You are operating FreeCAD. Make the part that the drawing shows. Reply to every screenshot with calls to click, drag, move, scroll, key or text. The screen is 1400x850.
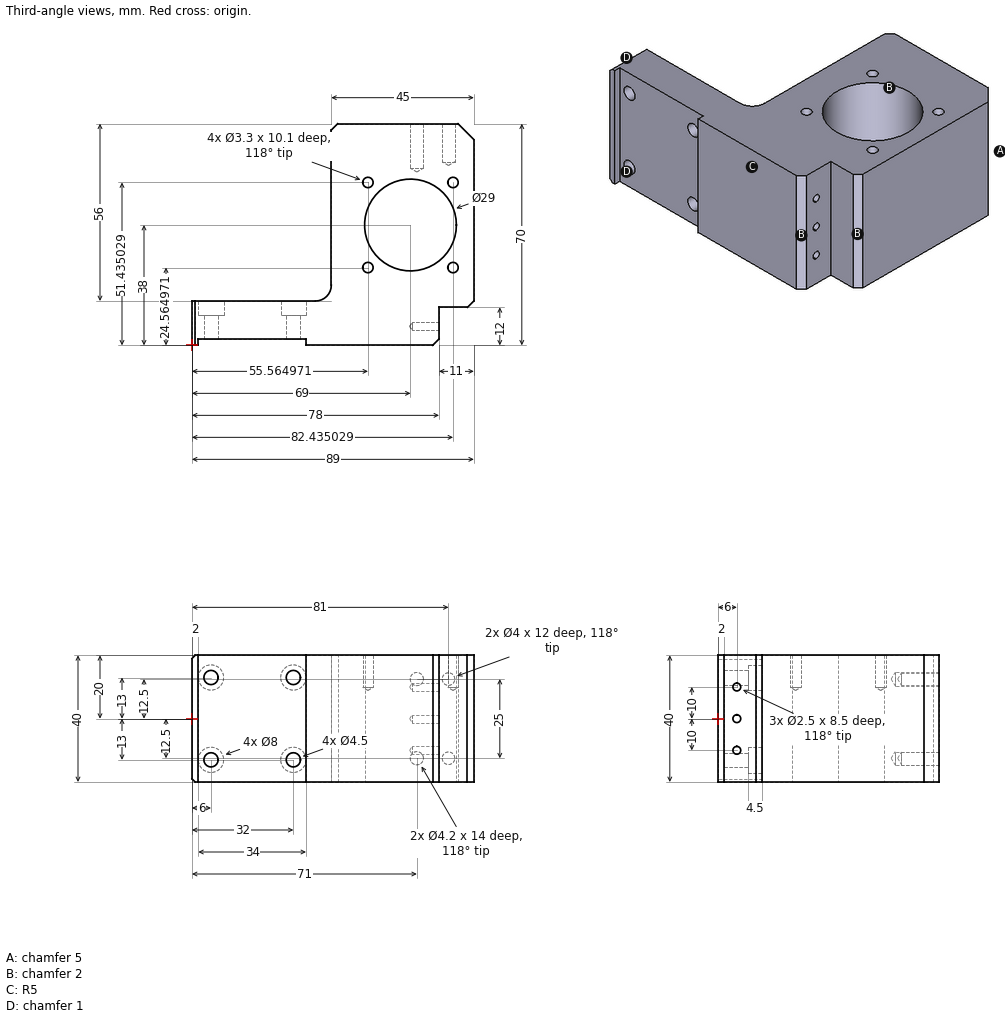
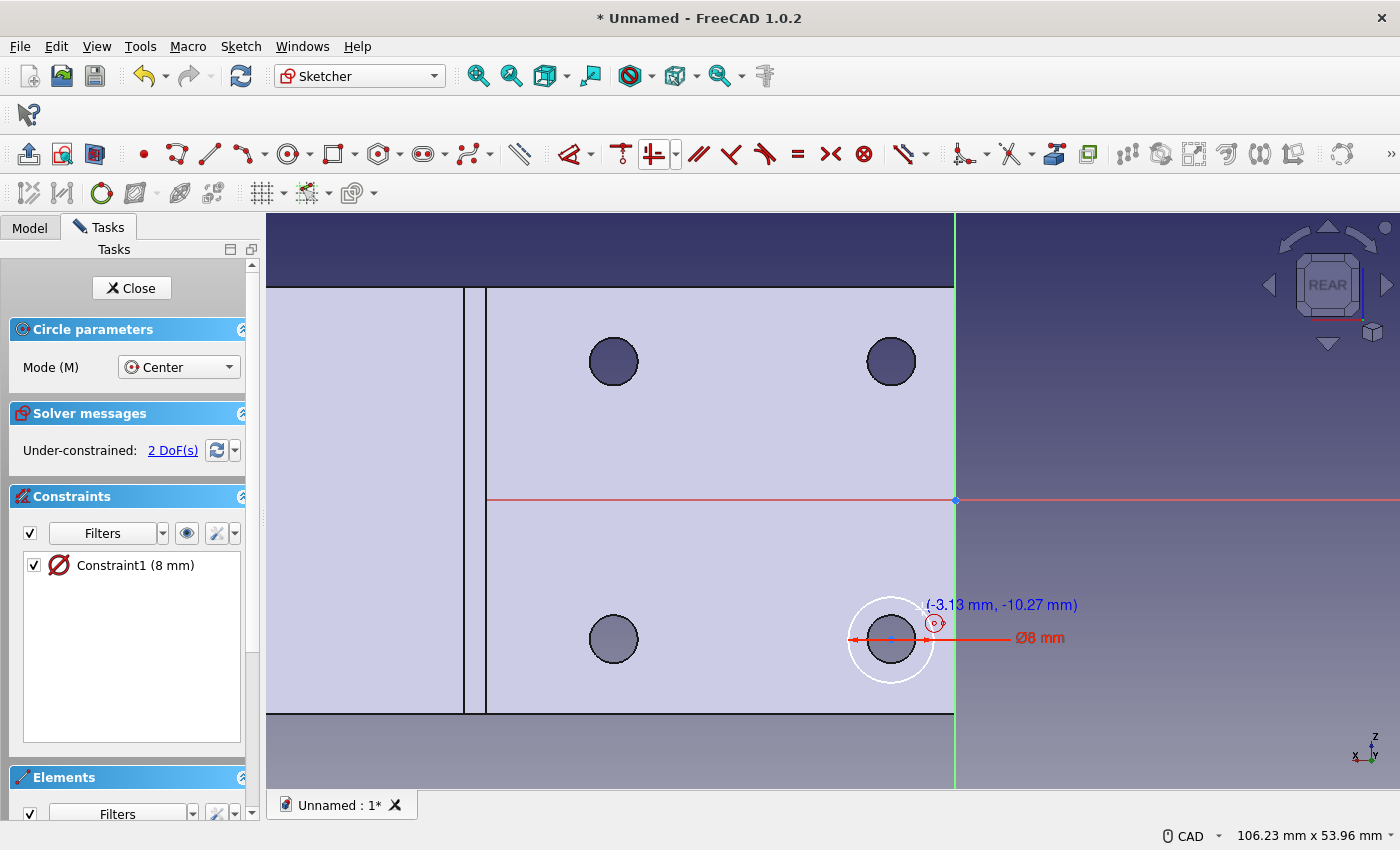
click(614, 639)
move(644, 609)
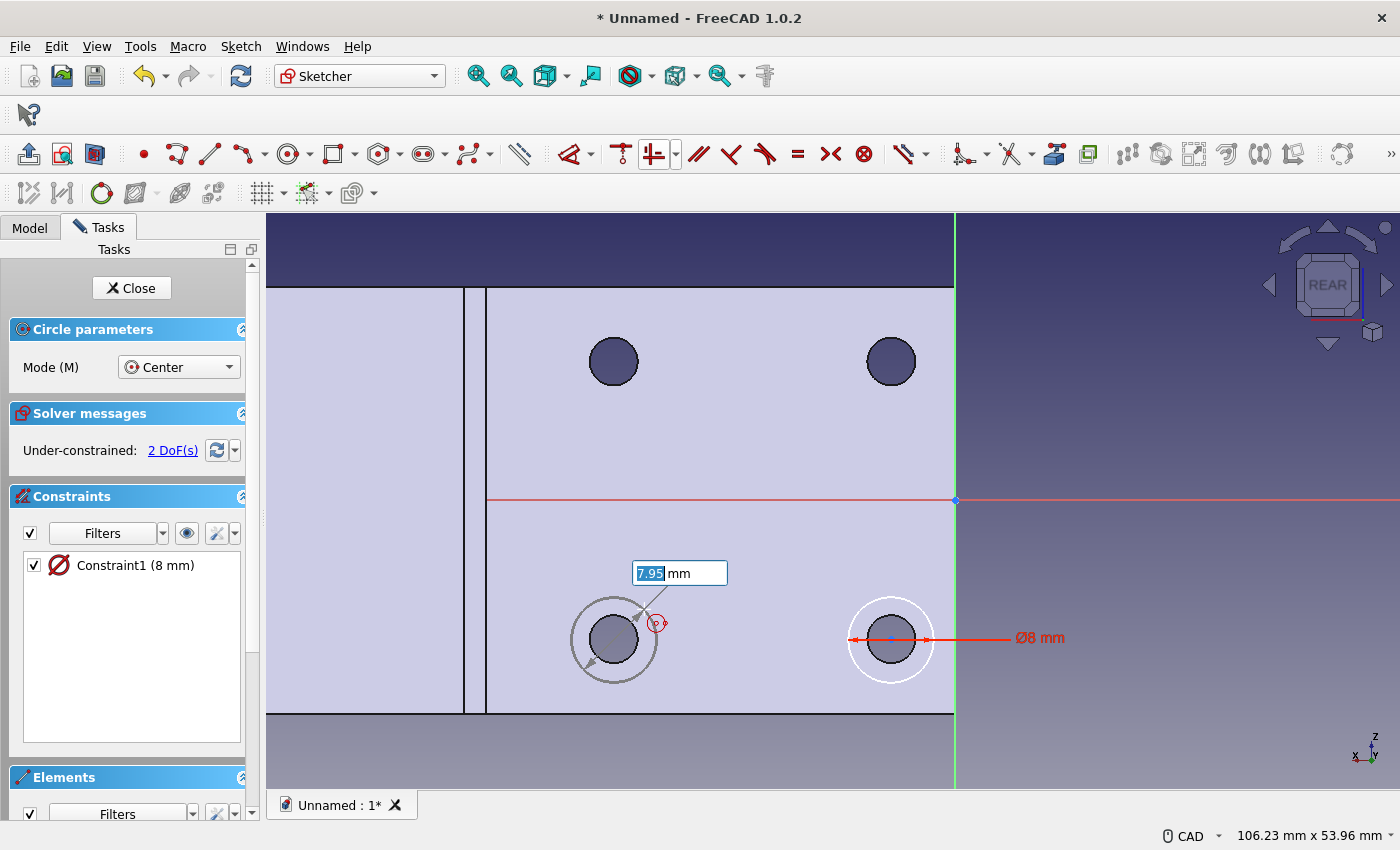
text(8)
key(Return)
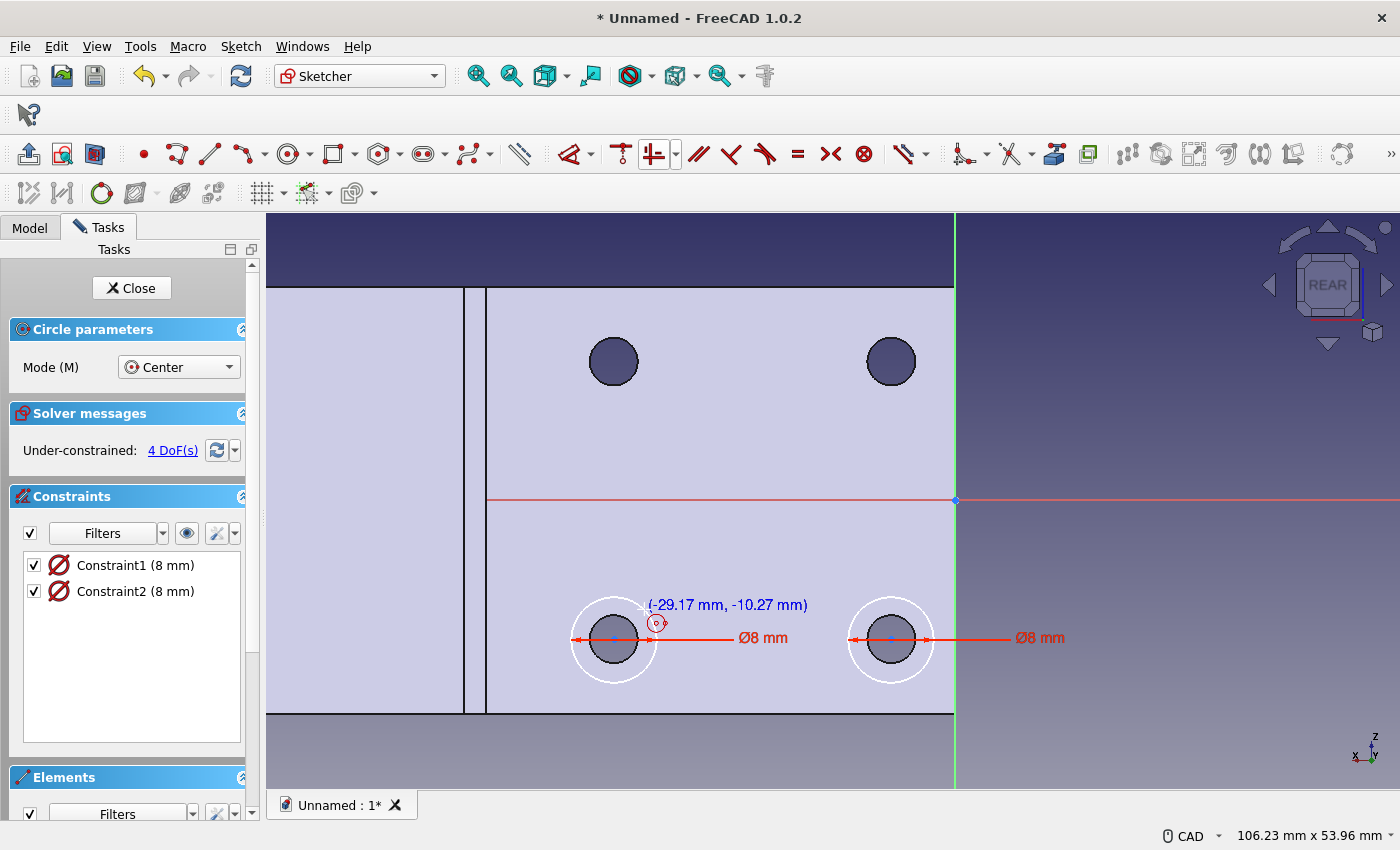
click(614, 362)
move(644, 331)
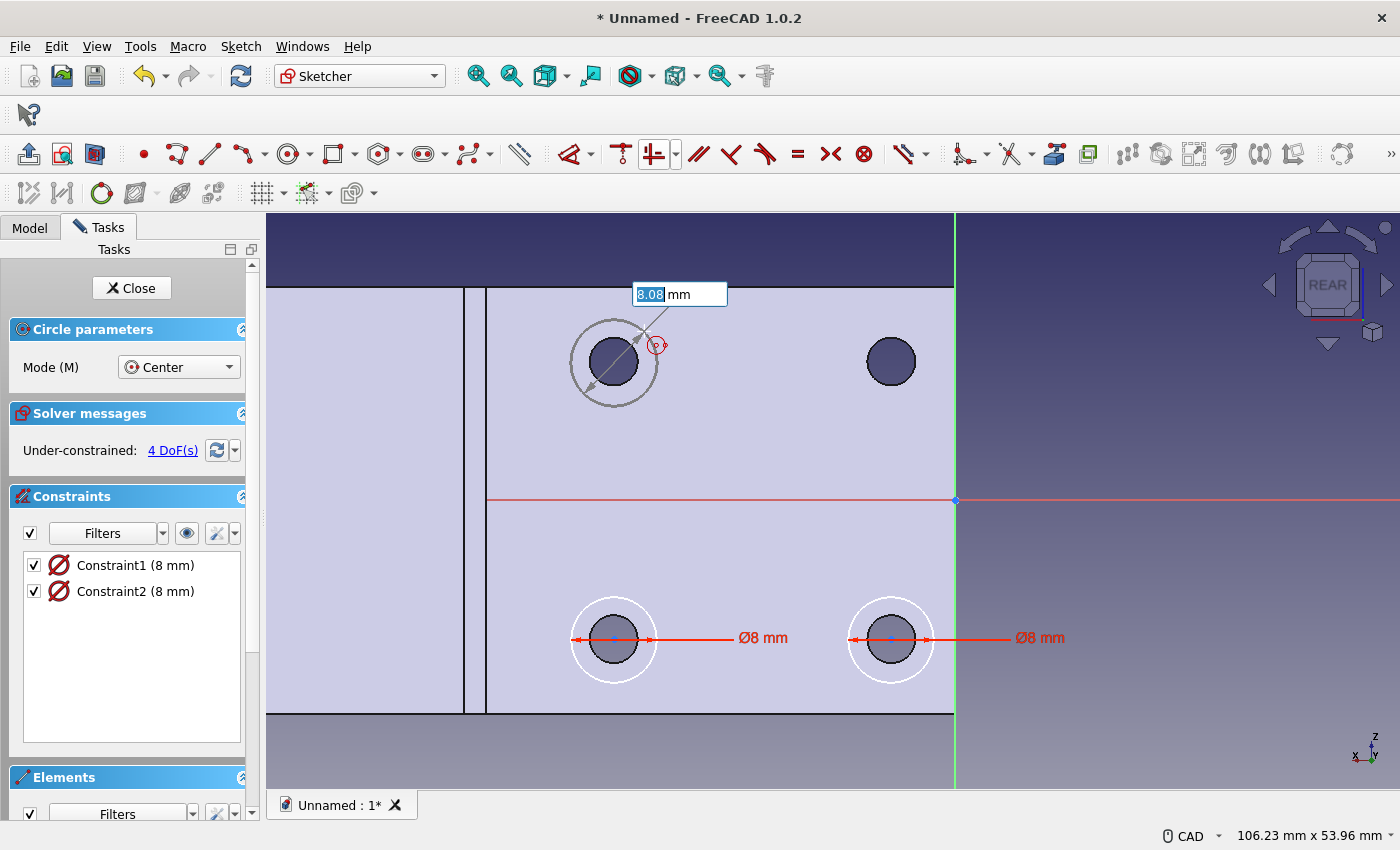
text(8)
key(Return)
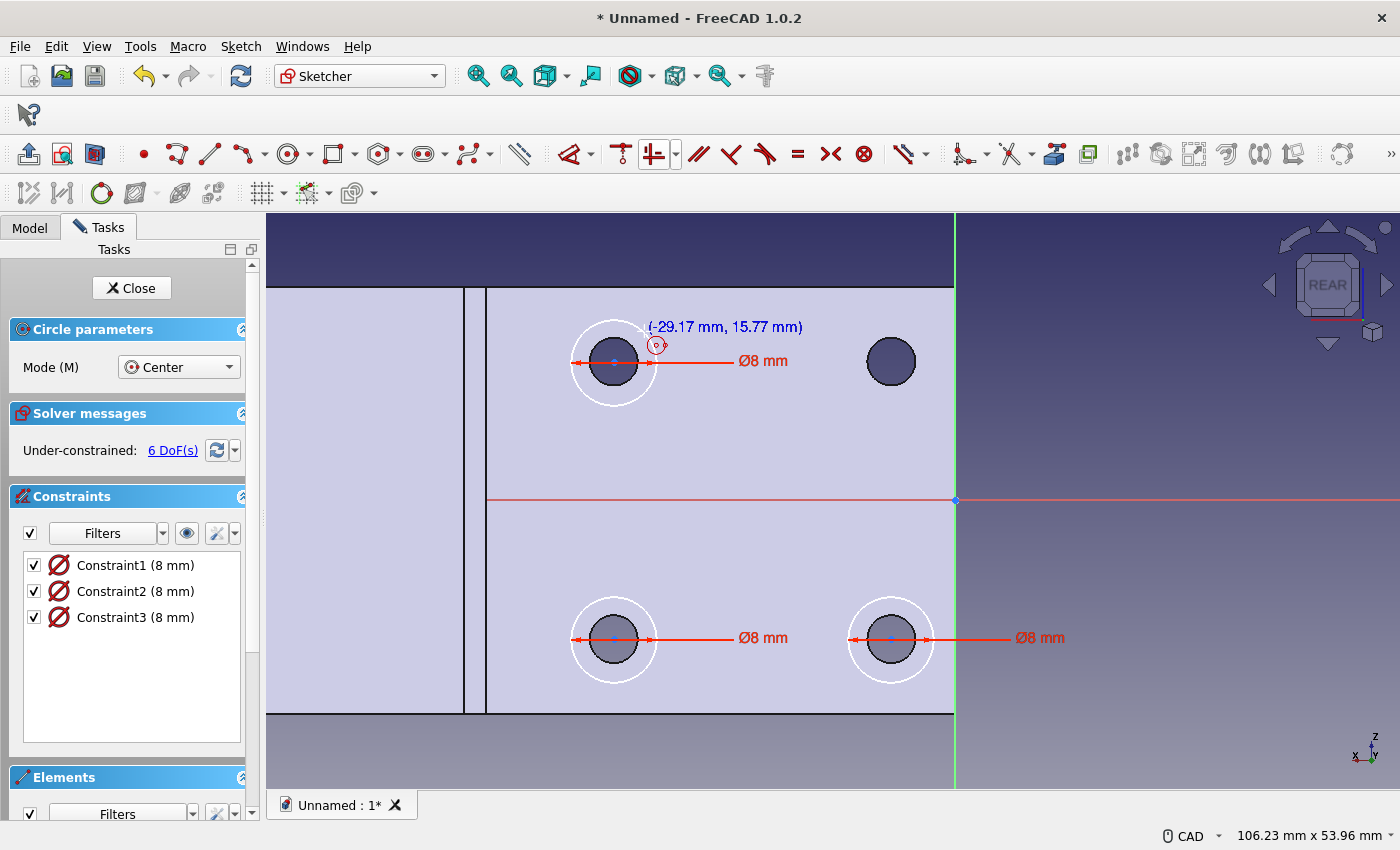
click(891, 362)
move(922, 331)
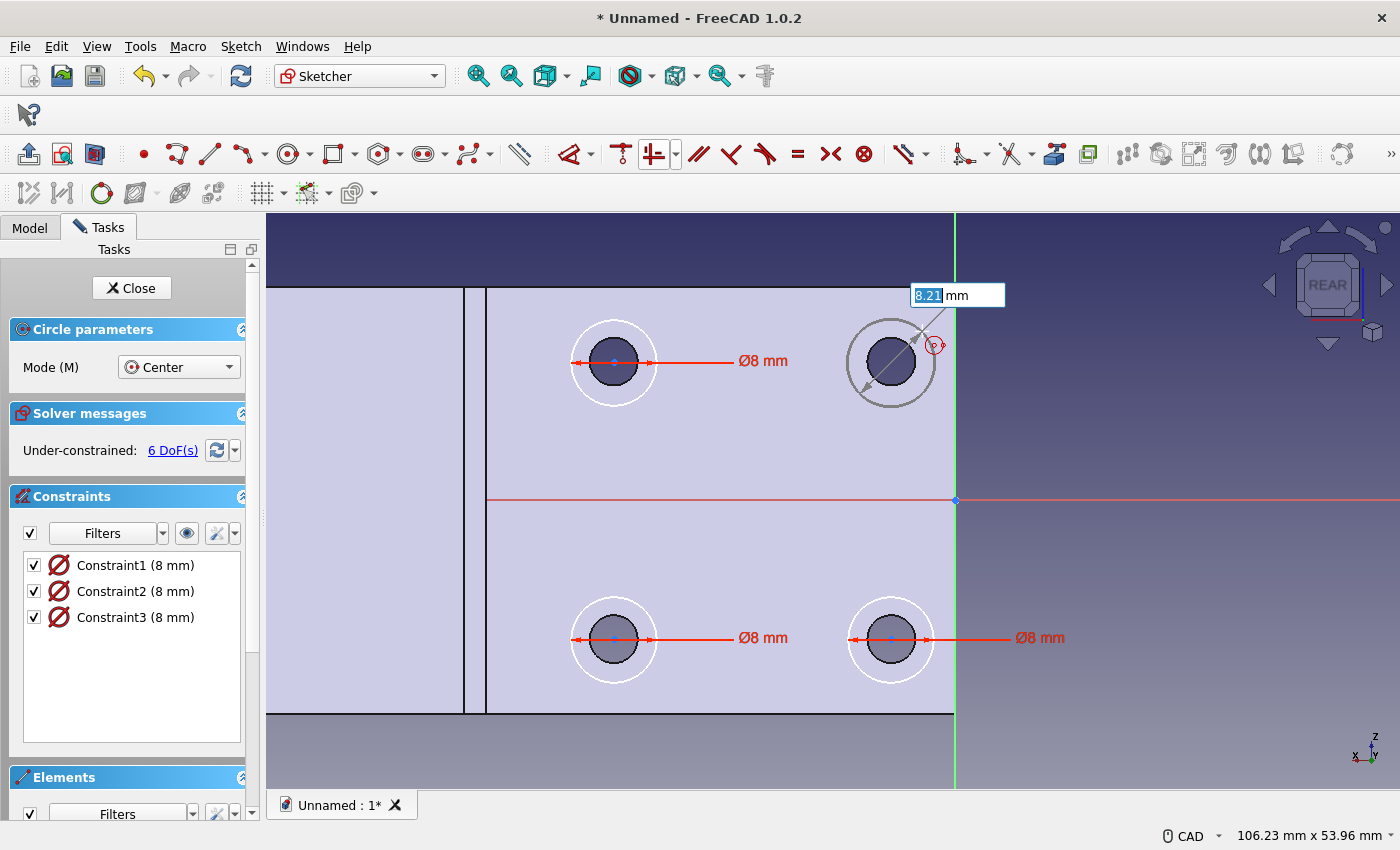
text(8)
key(Return)
key(Escape)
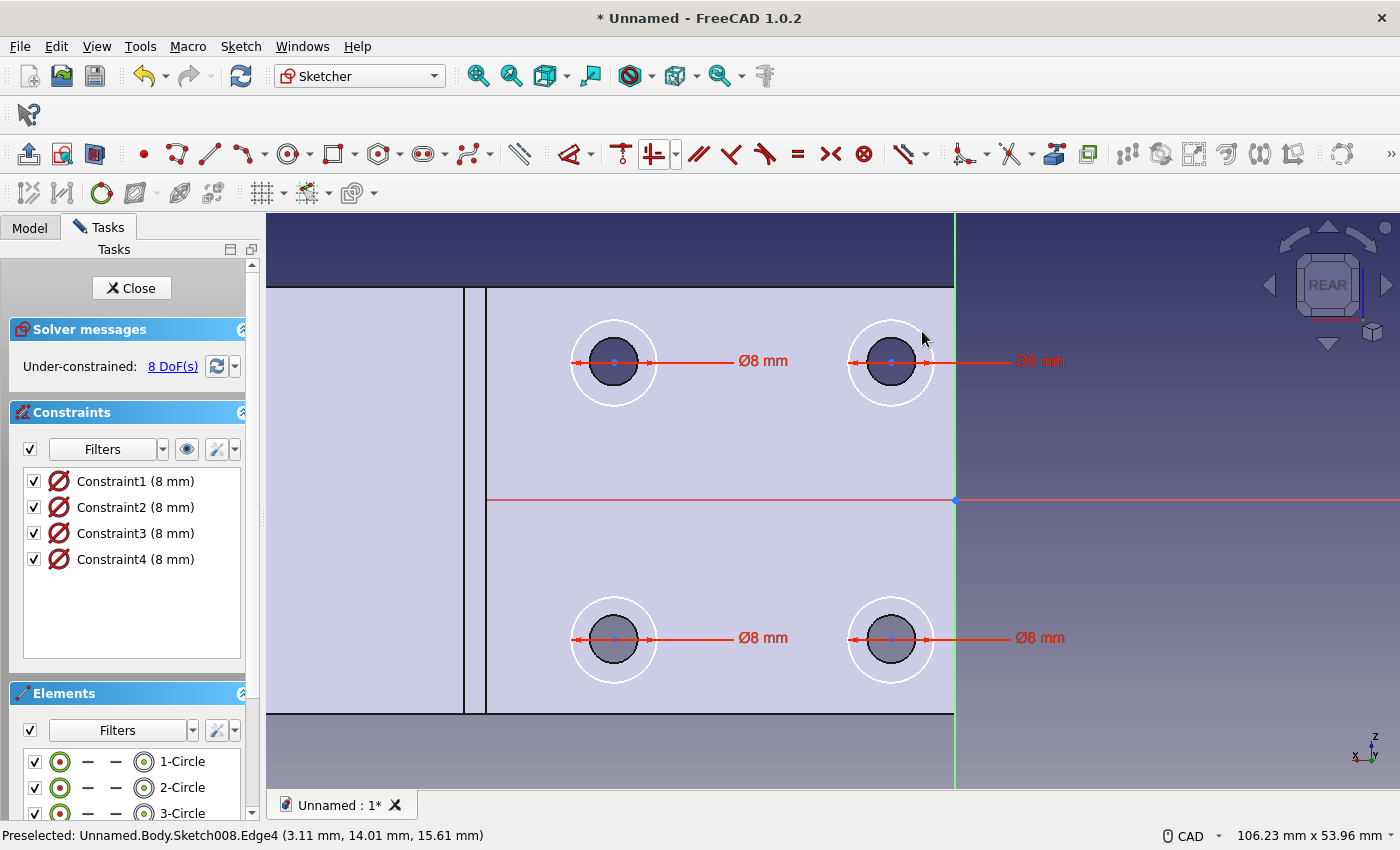
click(891, 640)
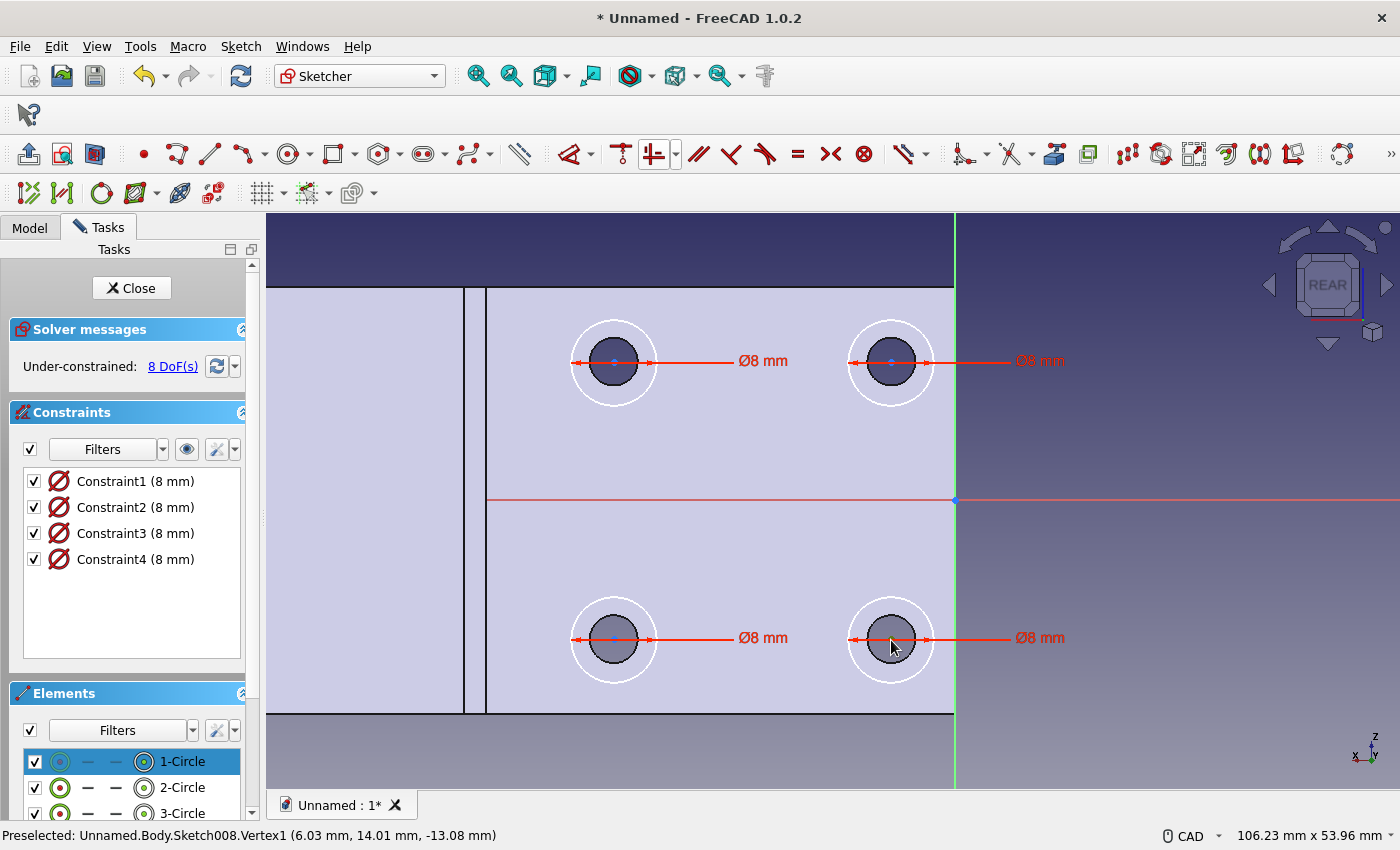
click(614, 640)